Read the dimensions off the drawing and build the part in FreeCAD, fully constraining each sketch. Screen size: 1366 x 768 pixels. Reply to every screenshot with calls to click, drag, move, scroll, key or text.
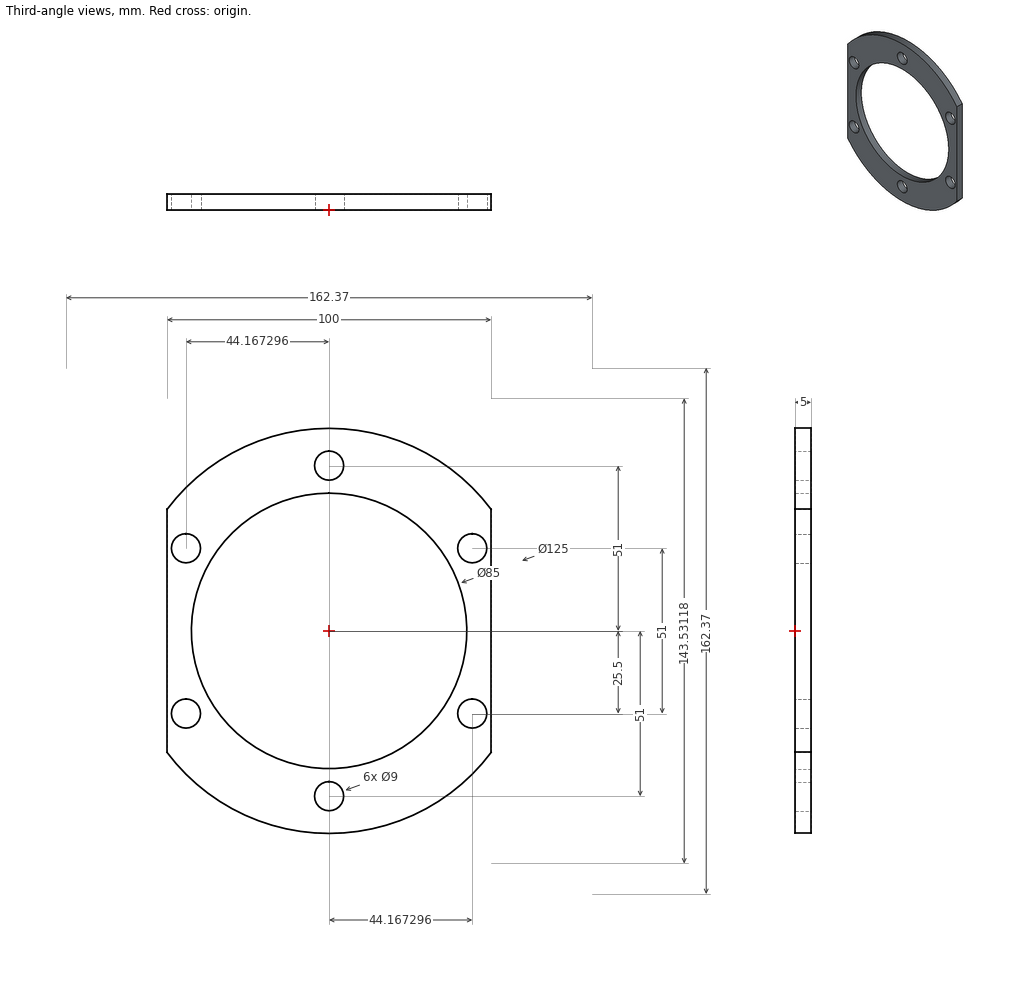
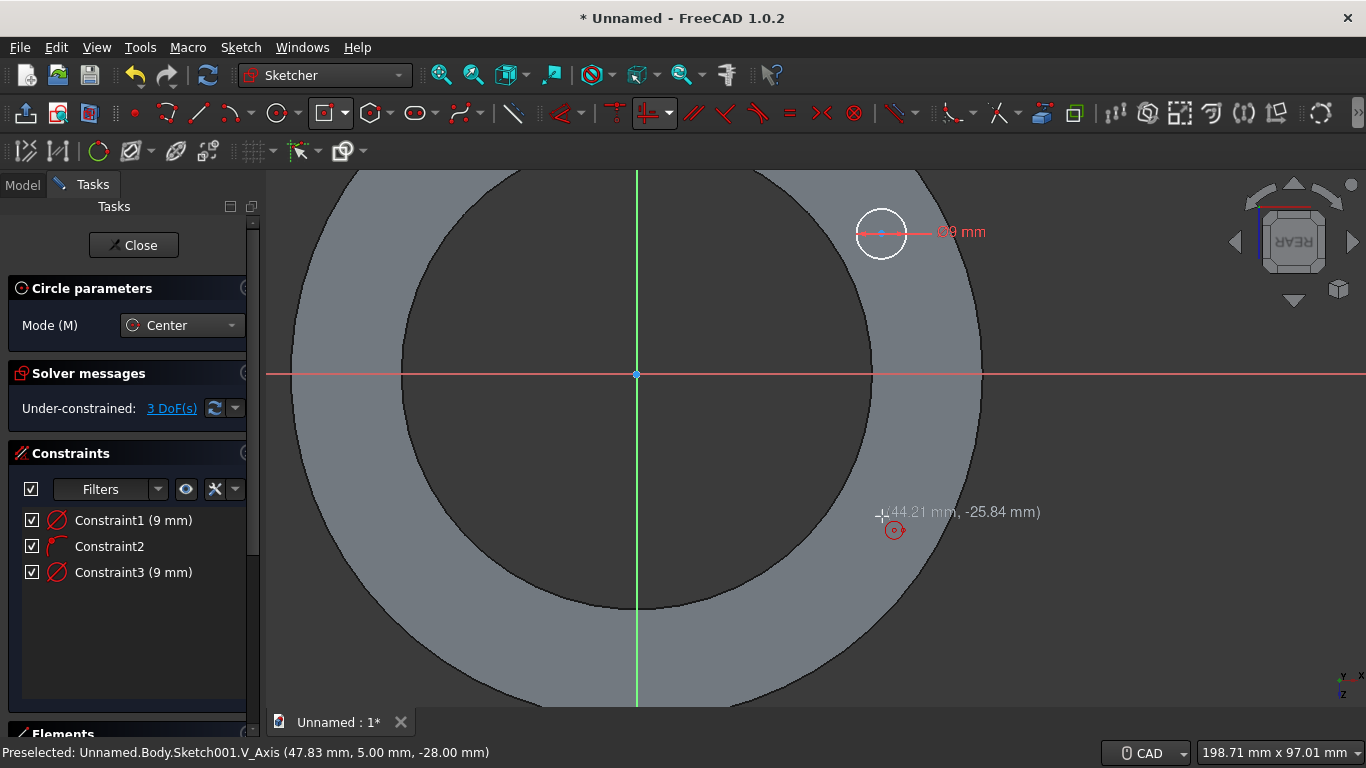
click(881, 515)
move(899, 498)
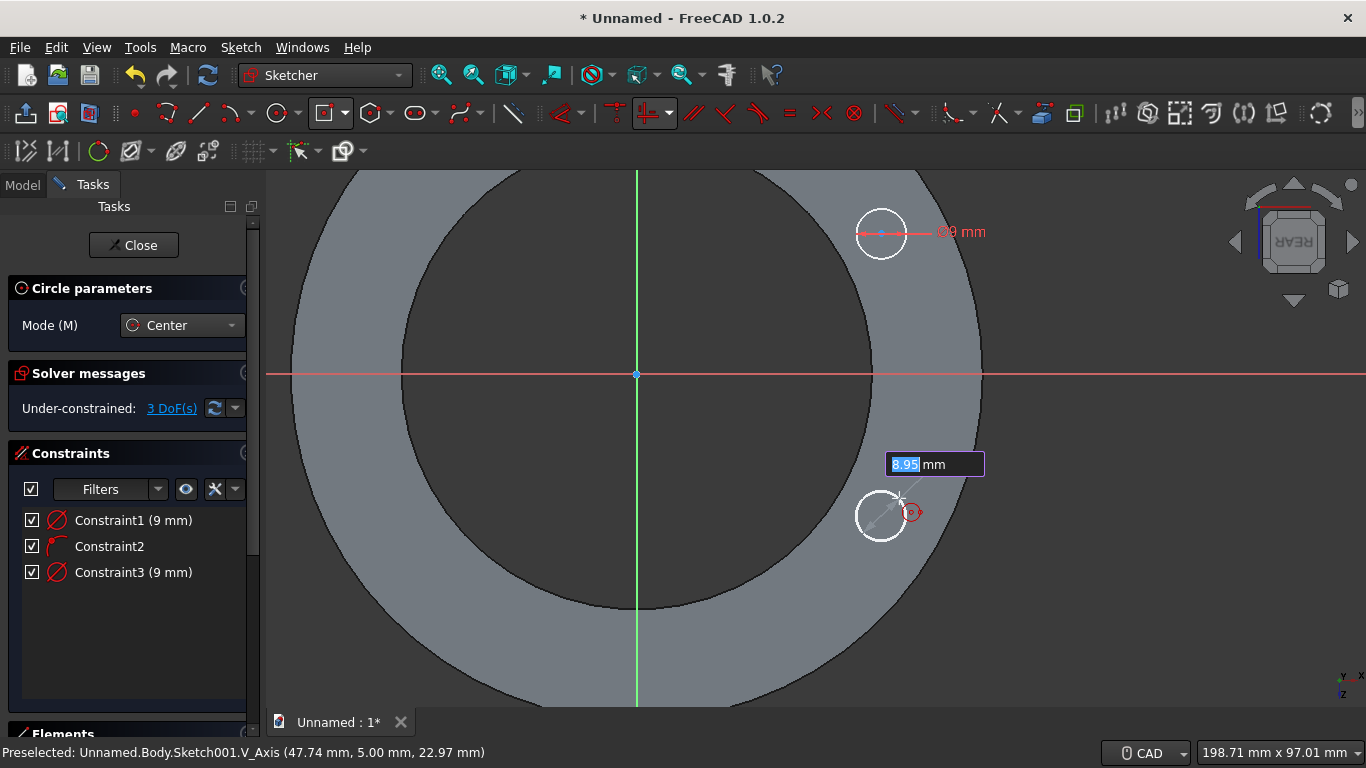
text(9)
key(Return)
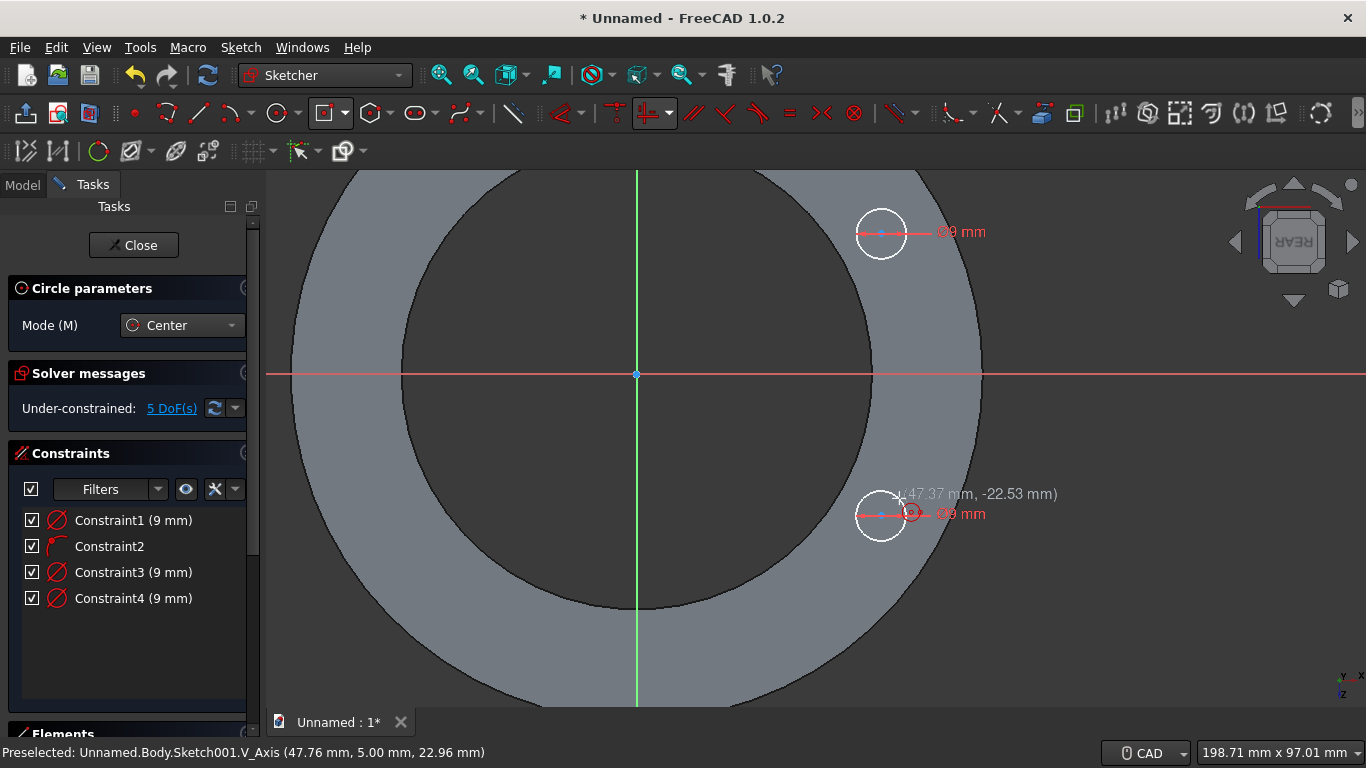
click(637, 657)
move(654, 639)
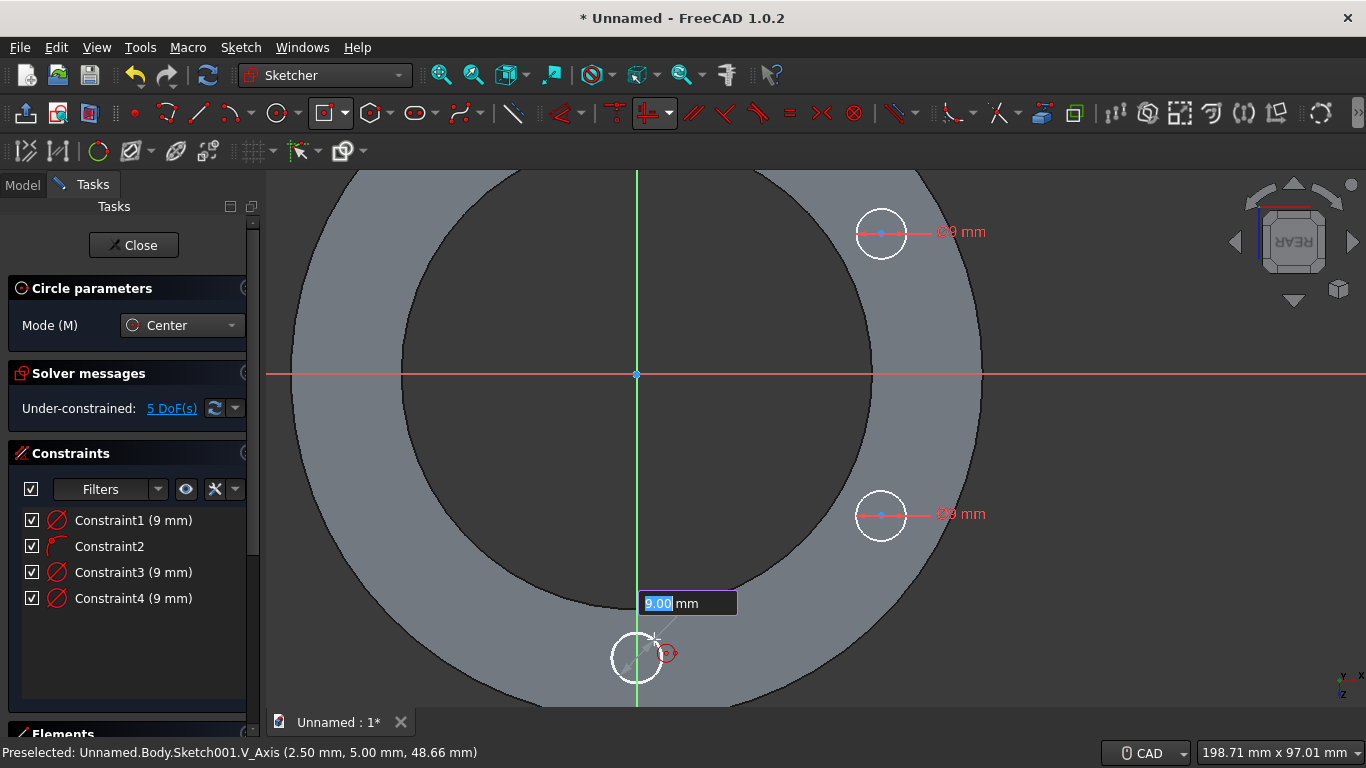
text(9)
key(Return)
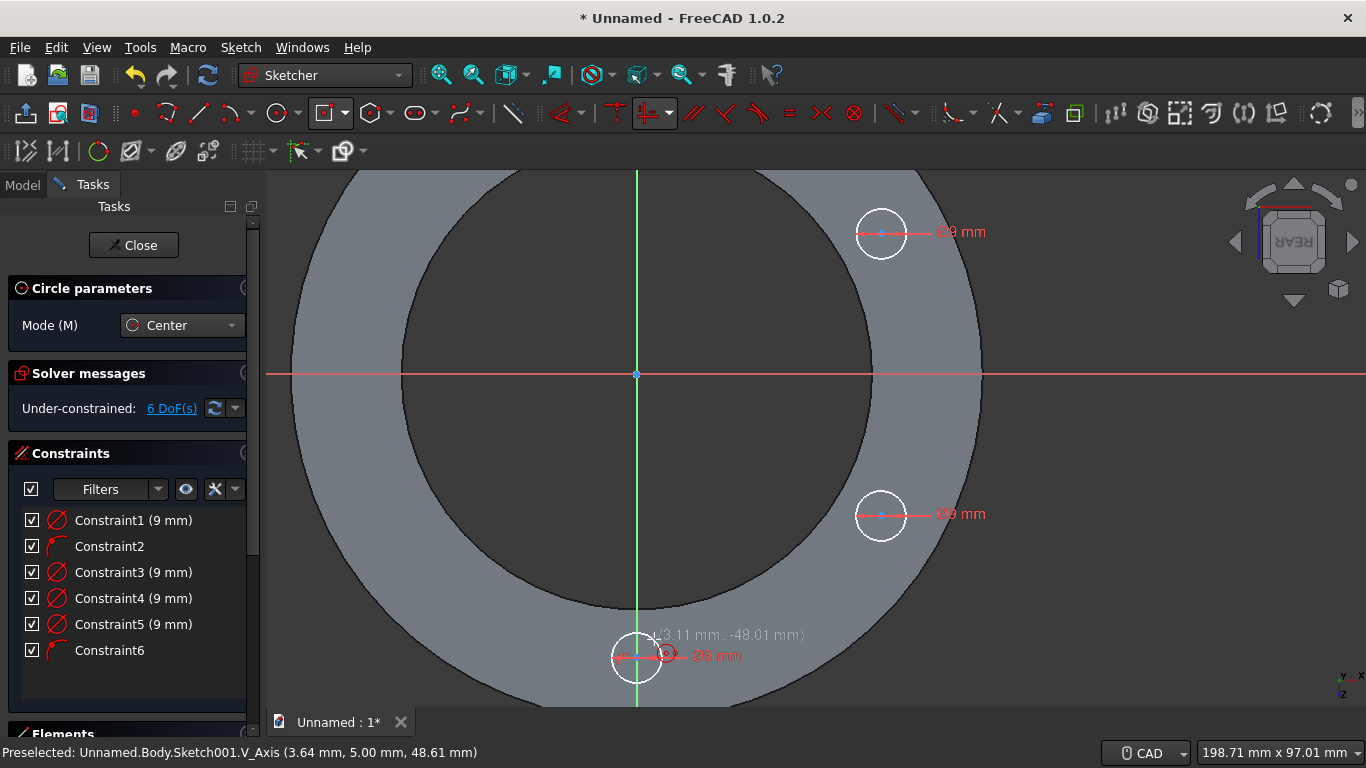
click(392, 515)
move(410, 498)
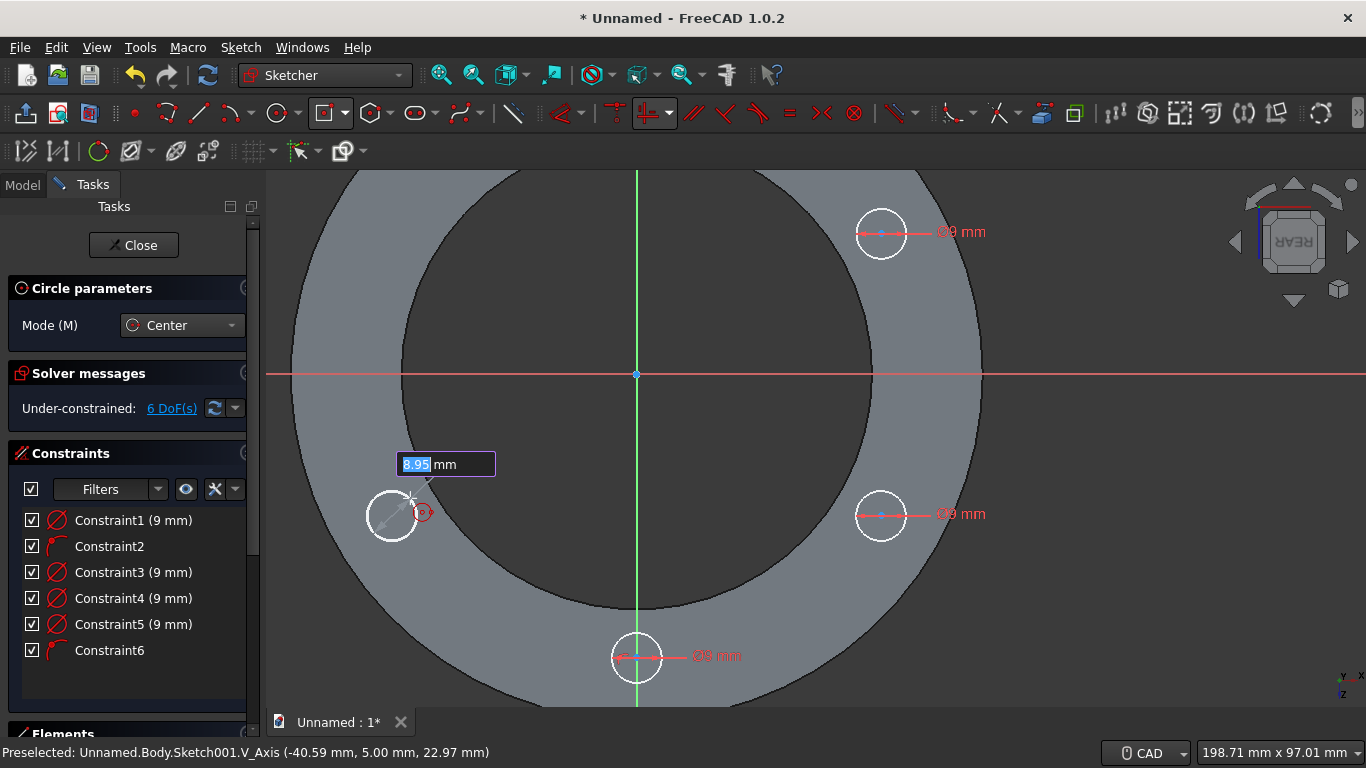
text(9)
key(Return)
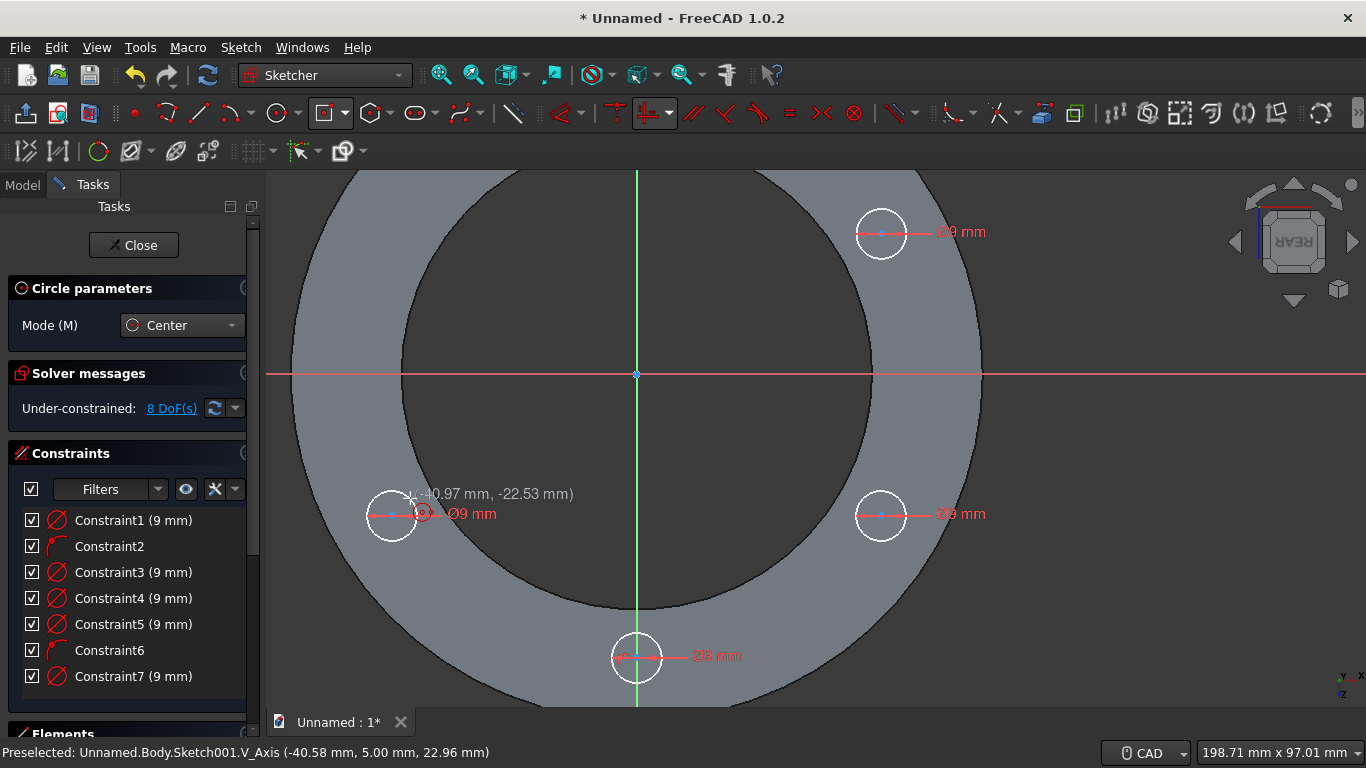
click(392, 233)
move(410, 215)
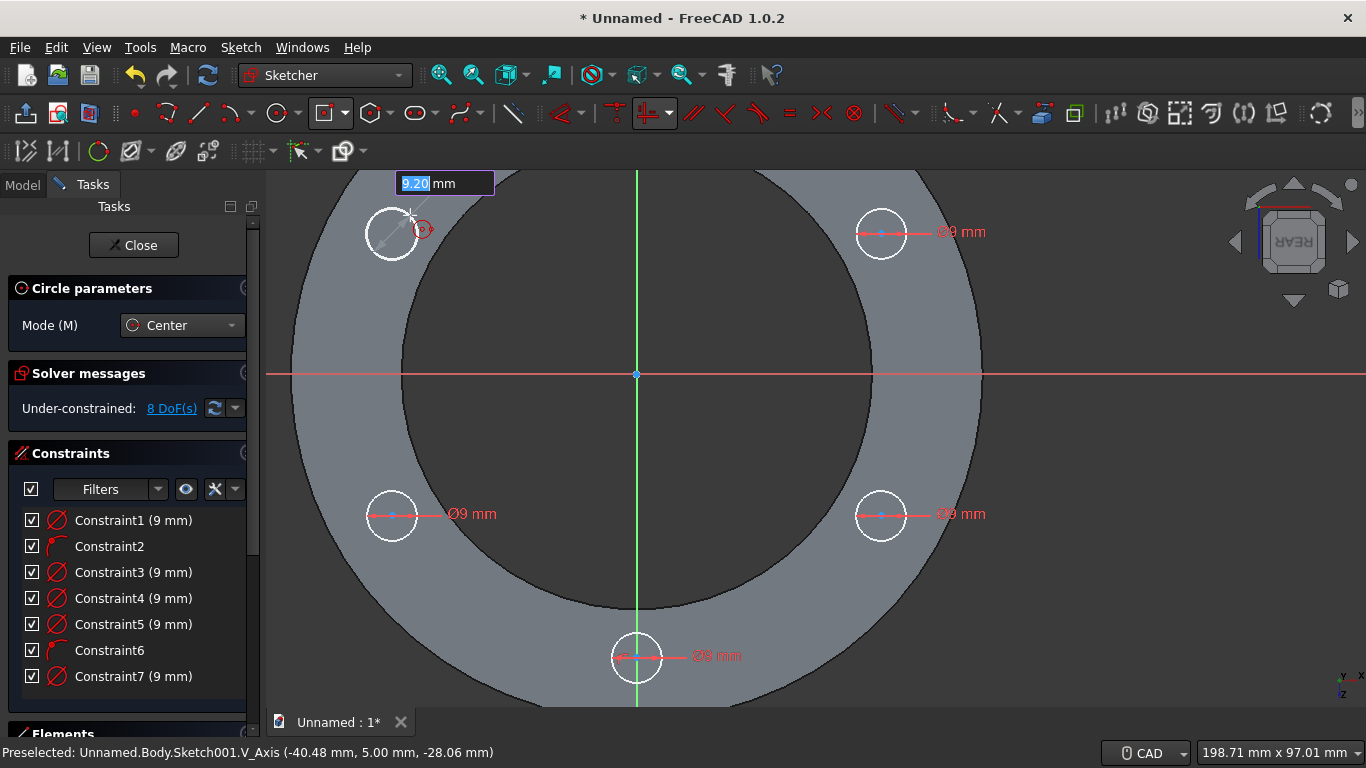
text(9)
key(Return)
key(Escape)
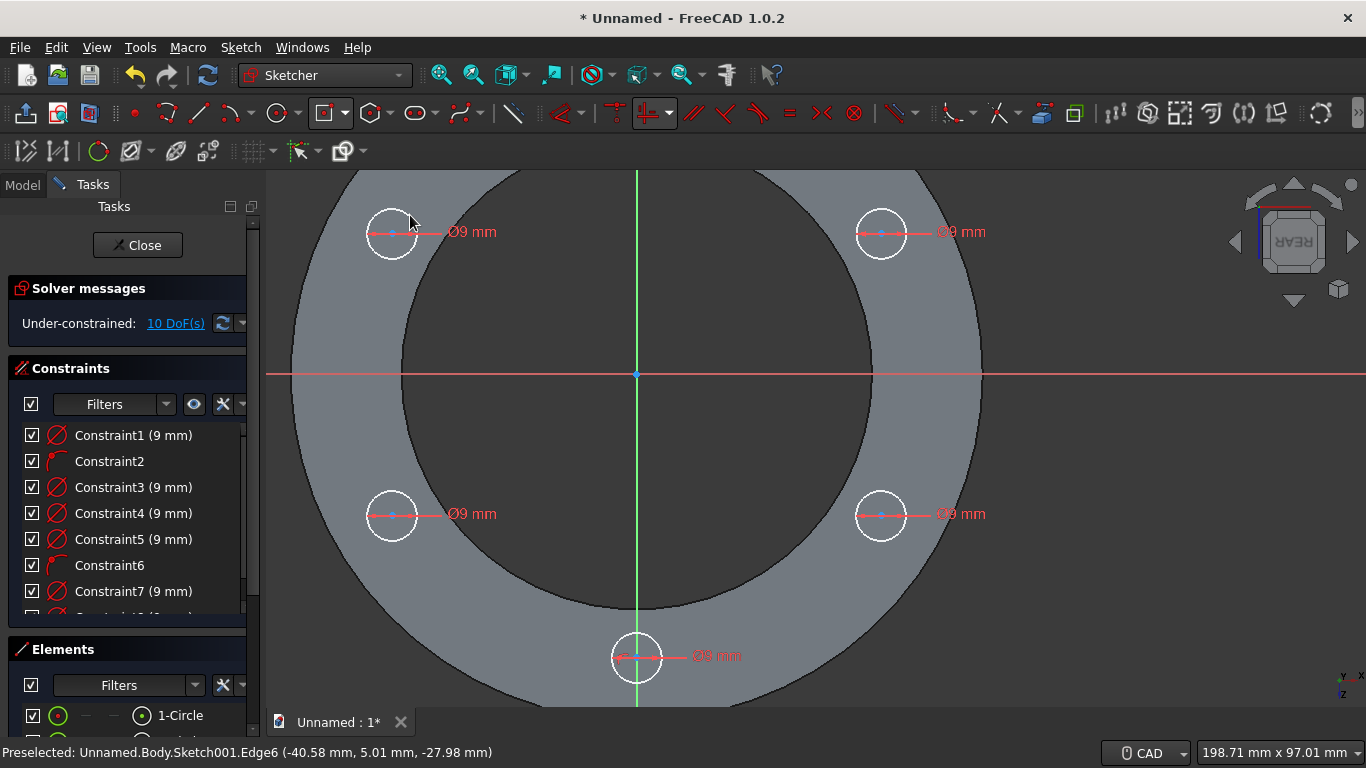
click(881, 234)